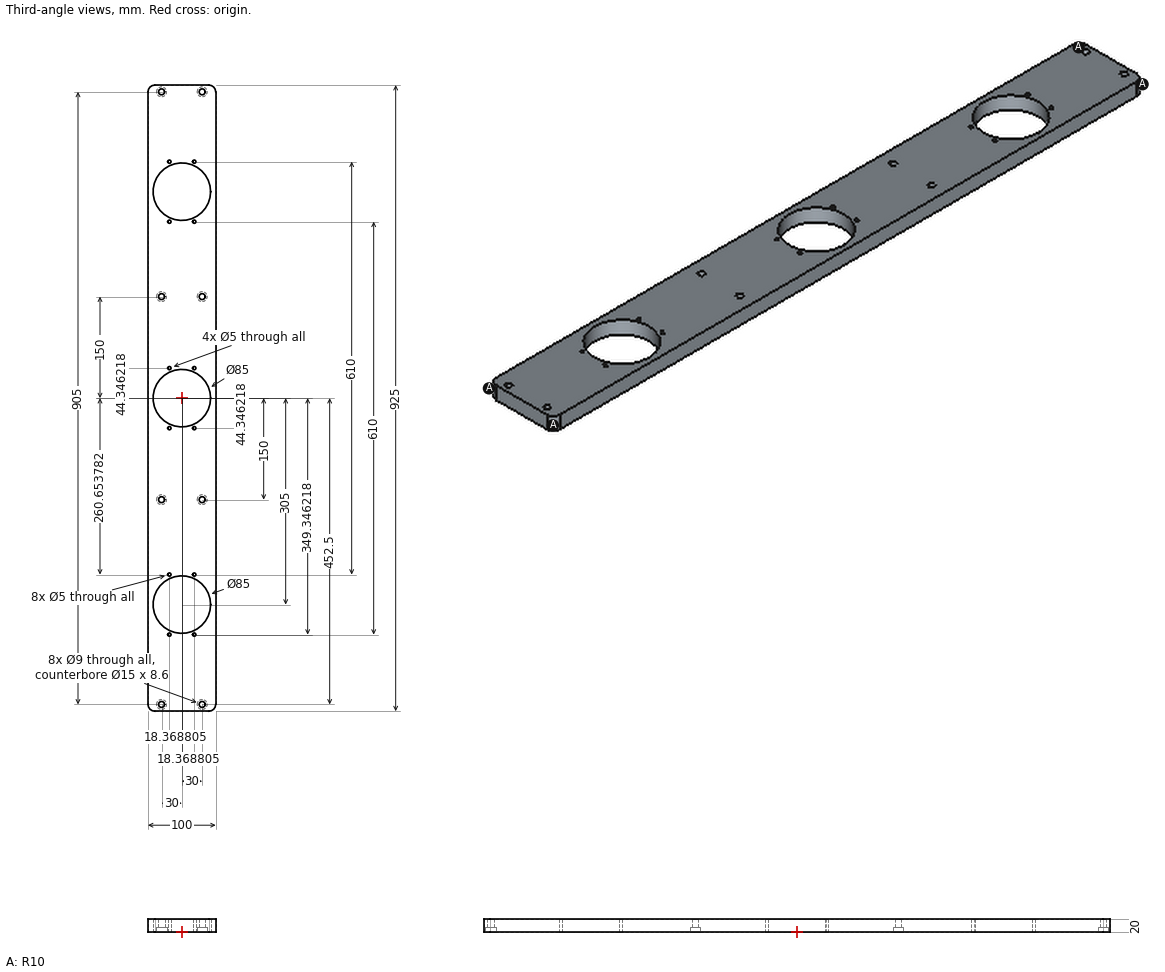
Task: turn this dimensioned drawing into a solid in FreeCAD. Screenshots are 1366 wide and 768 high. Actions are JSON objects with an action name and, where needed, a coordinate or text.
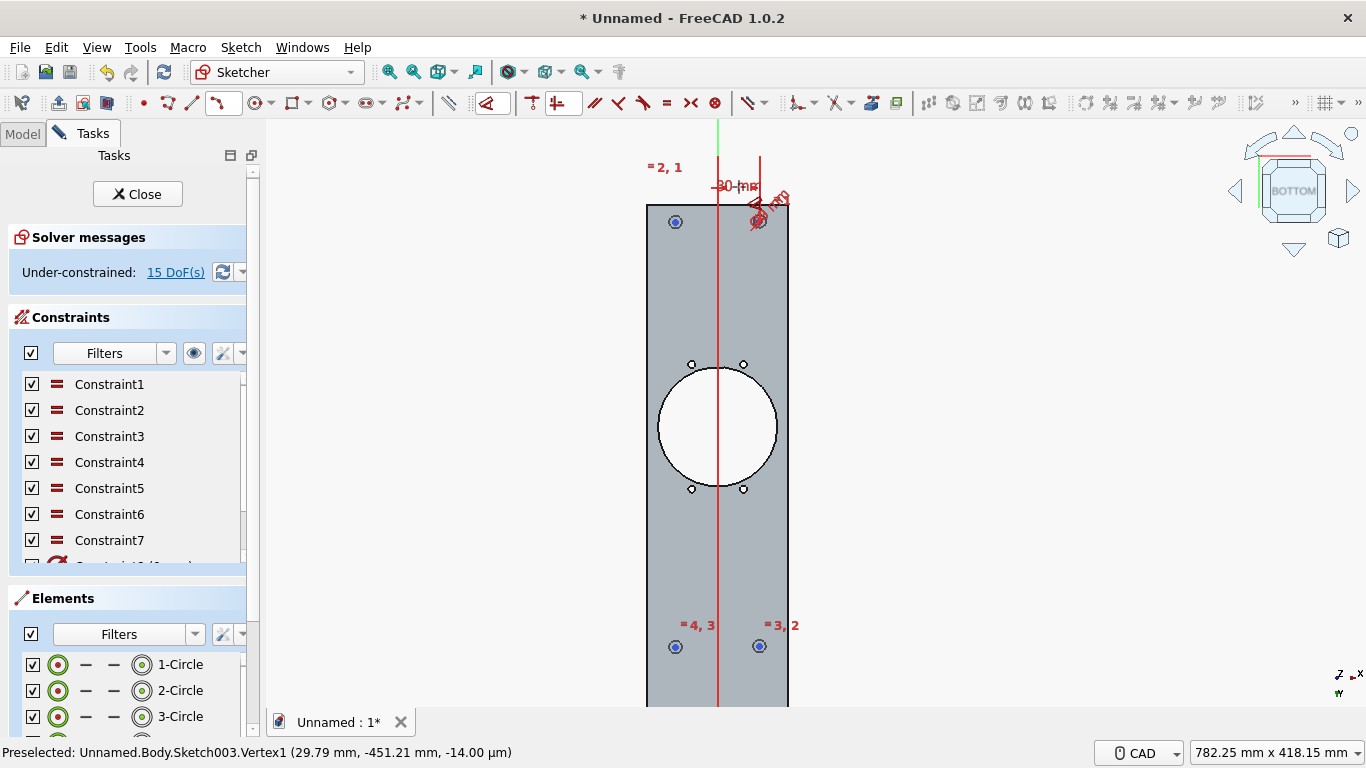
{"action": "left_click", "coordinate": [676, 222]}
{"action": "left_click", "coordinate": [697, 164]}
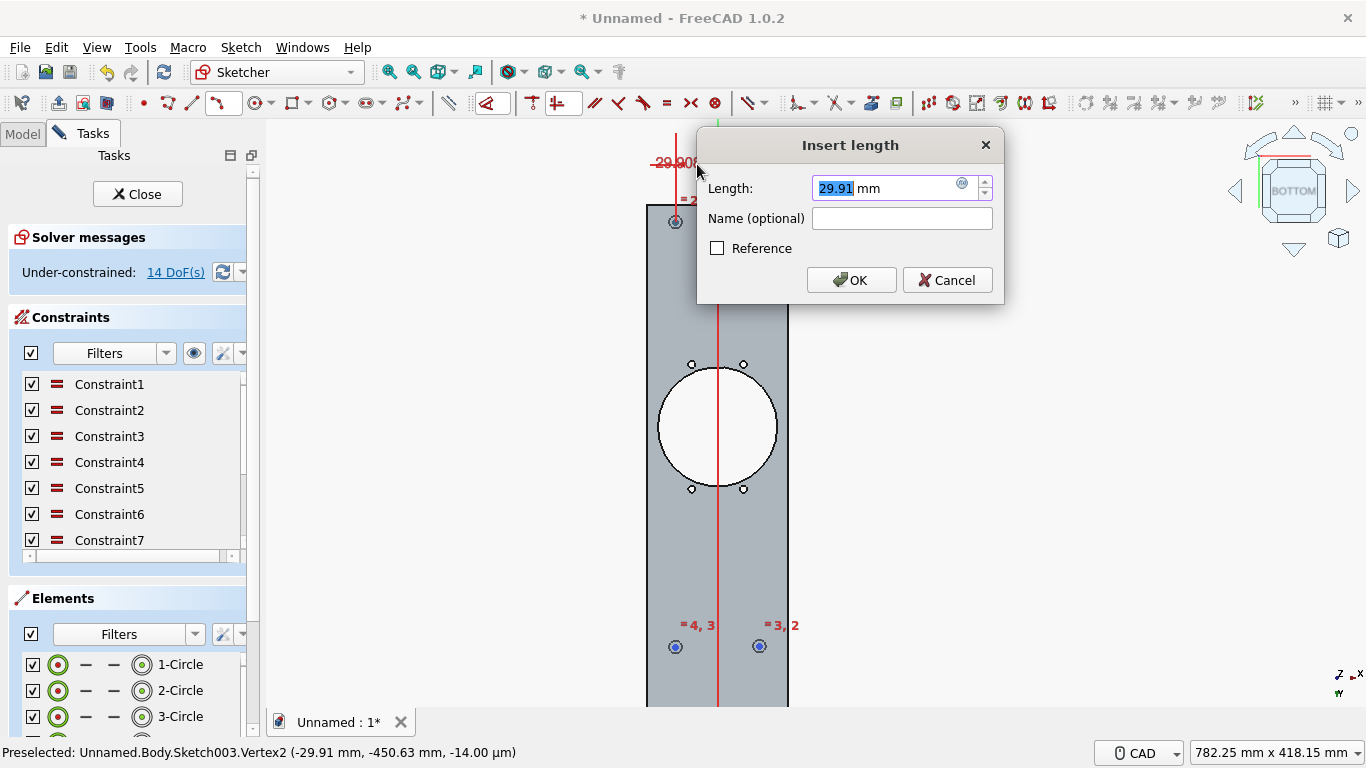
{"action": "type", "text": "30"}
{"action": "key", "text": "Return"}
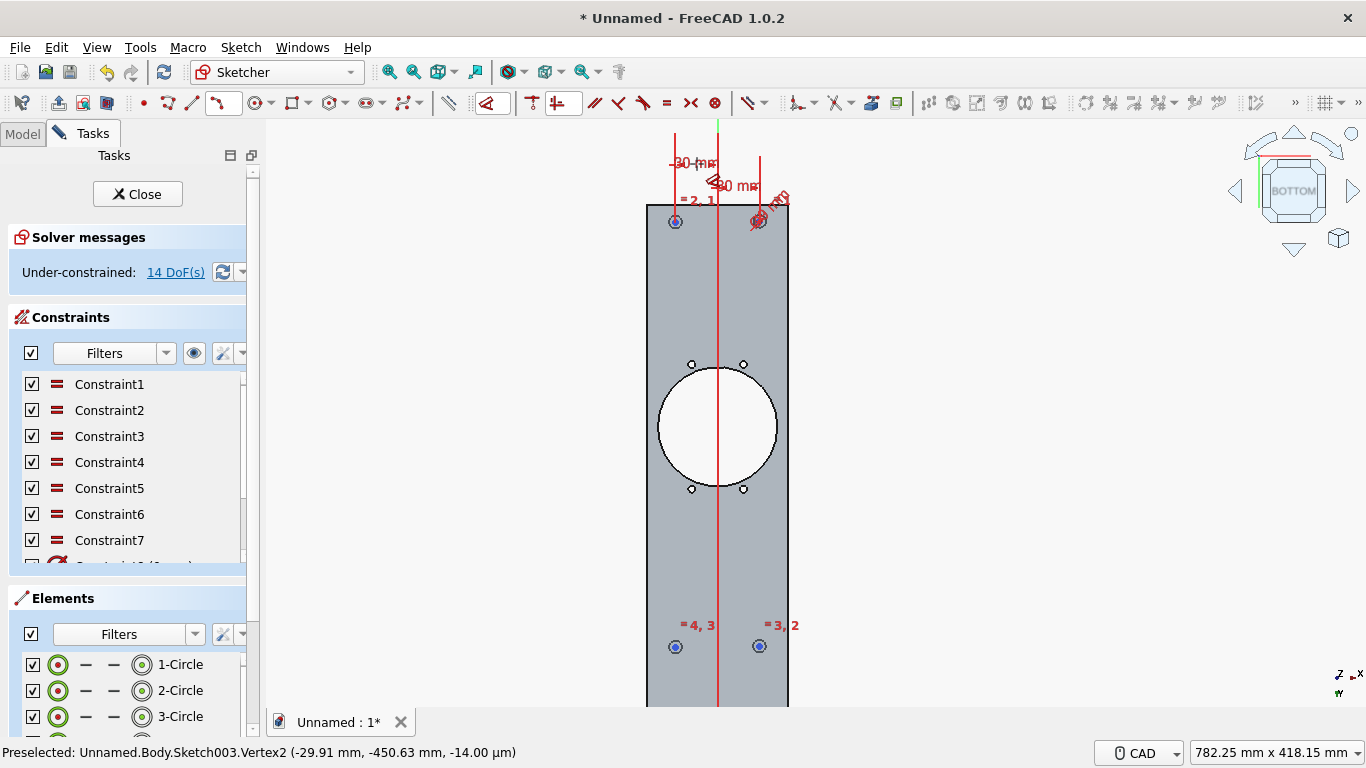
{"action": "left_click", "coordinate": [759, 646]}
{"action": "left_click", "coordinate": [739, 612]}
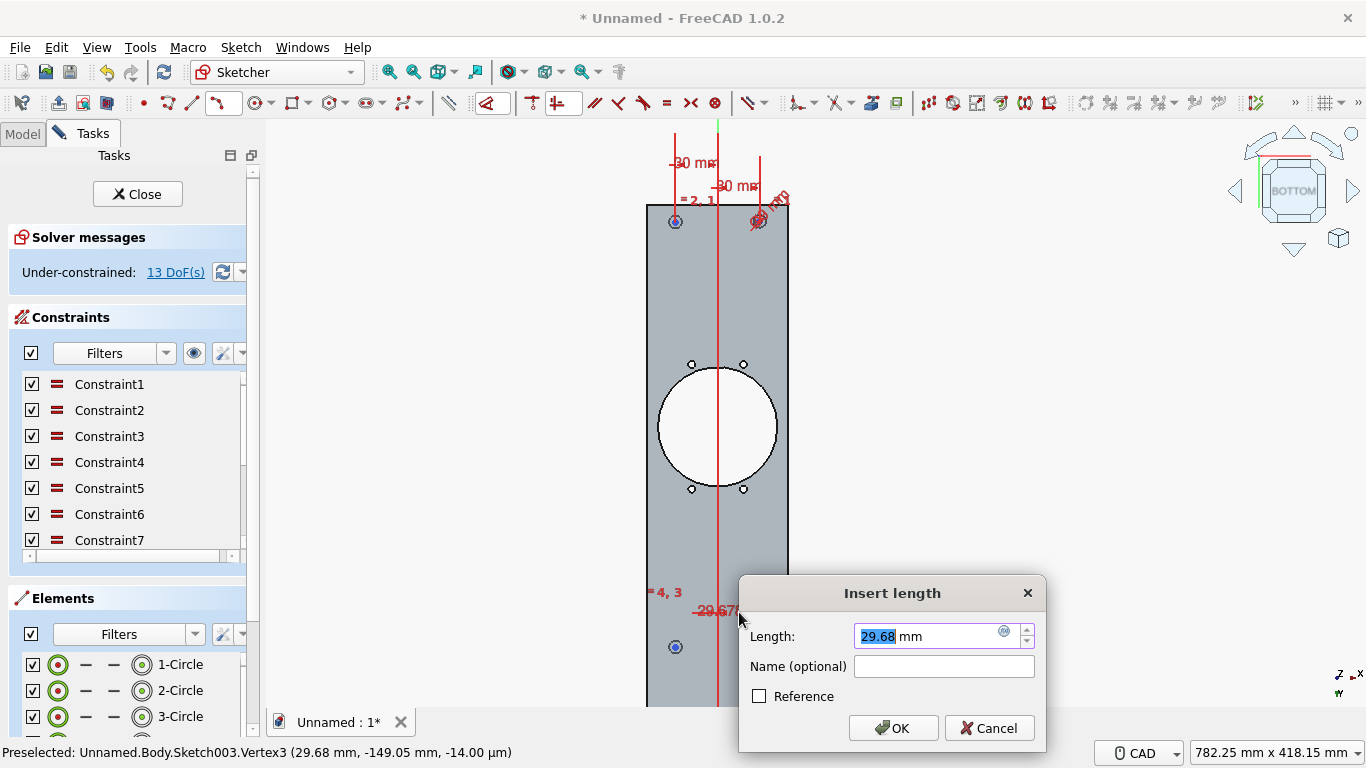
{"action": "type", "text": "30"}
{"action": "key", "text": "Return"}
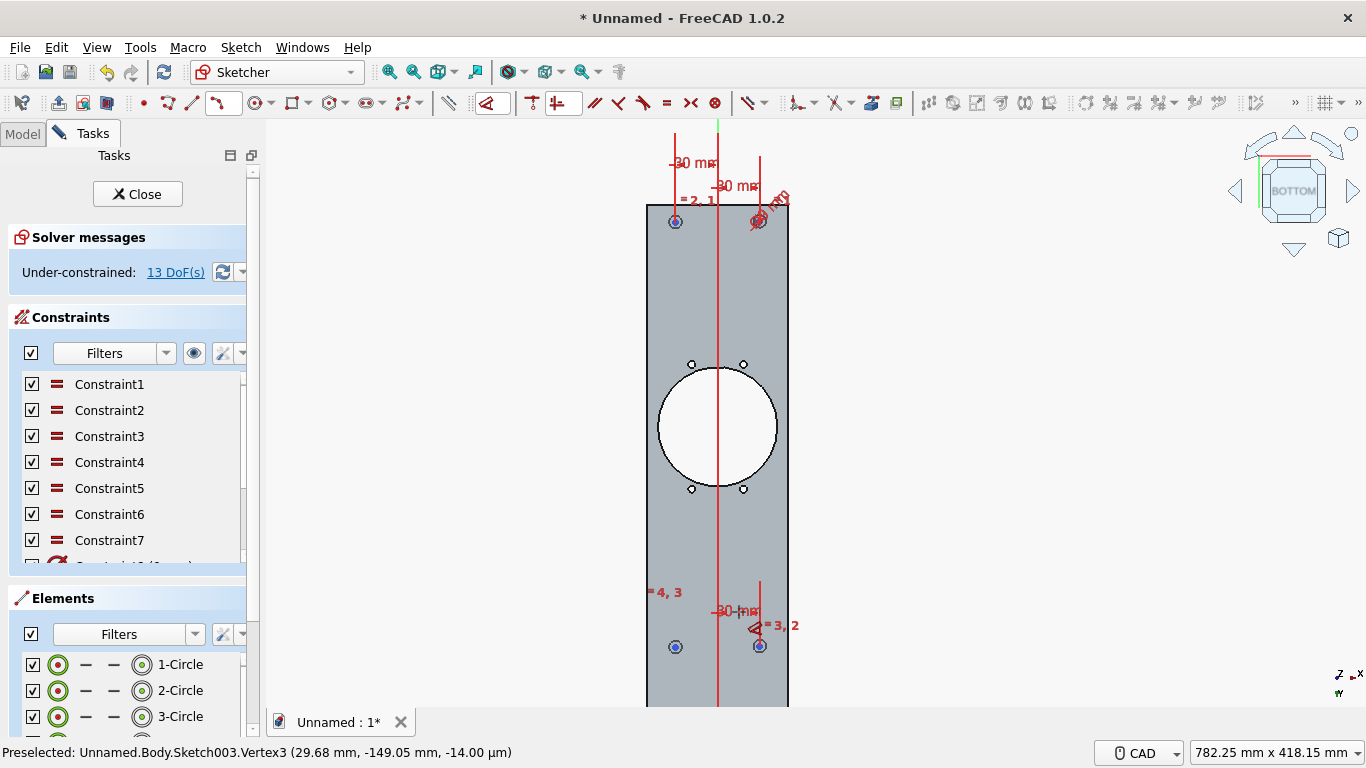
{"action": "left_click", "coordinate": [676, 647]}
{"action": "left_click", "coordinate": [697, 589]}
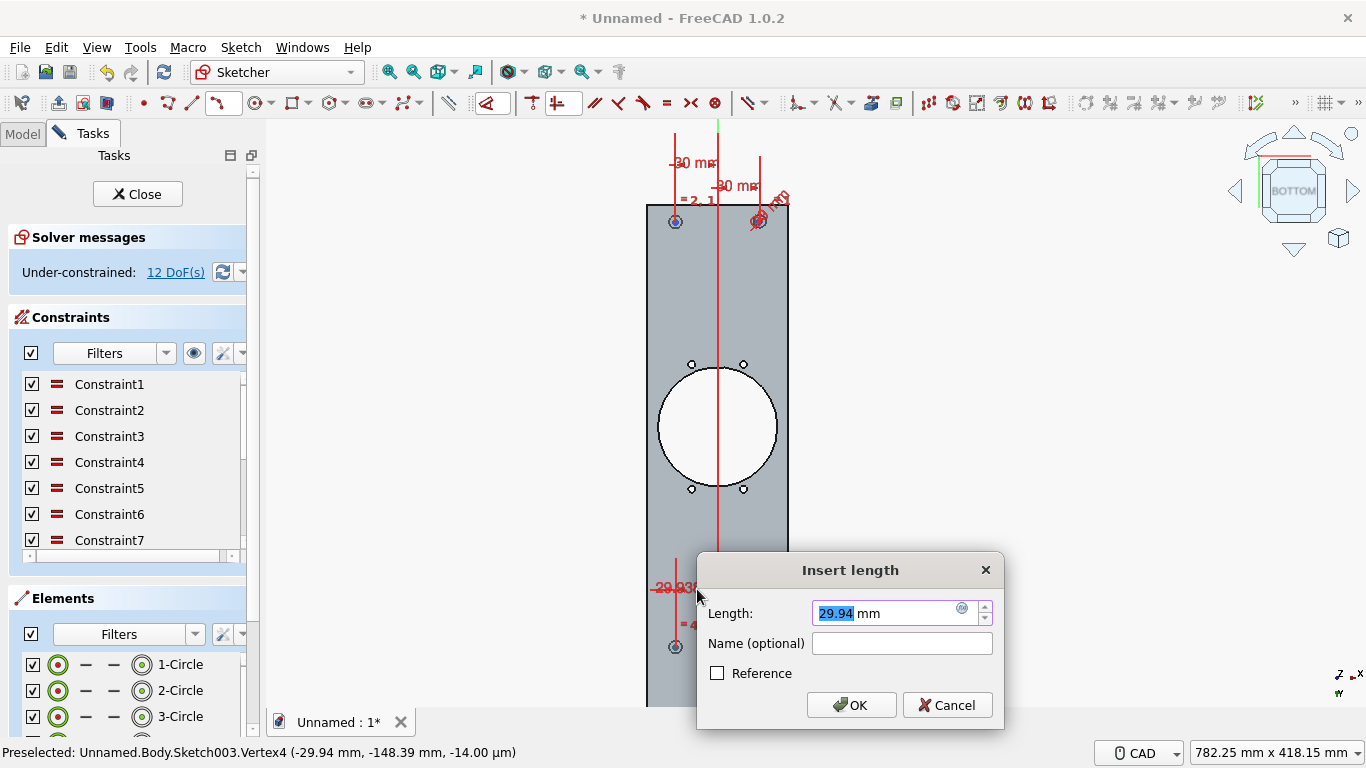
{"action": "type", "text": "30"}
{"action": "key", "text": "Return"}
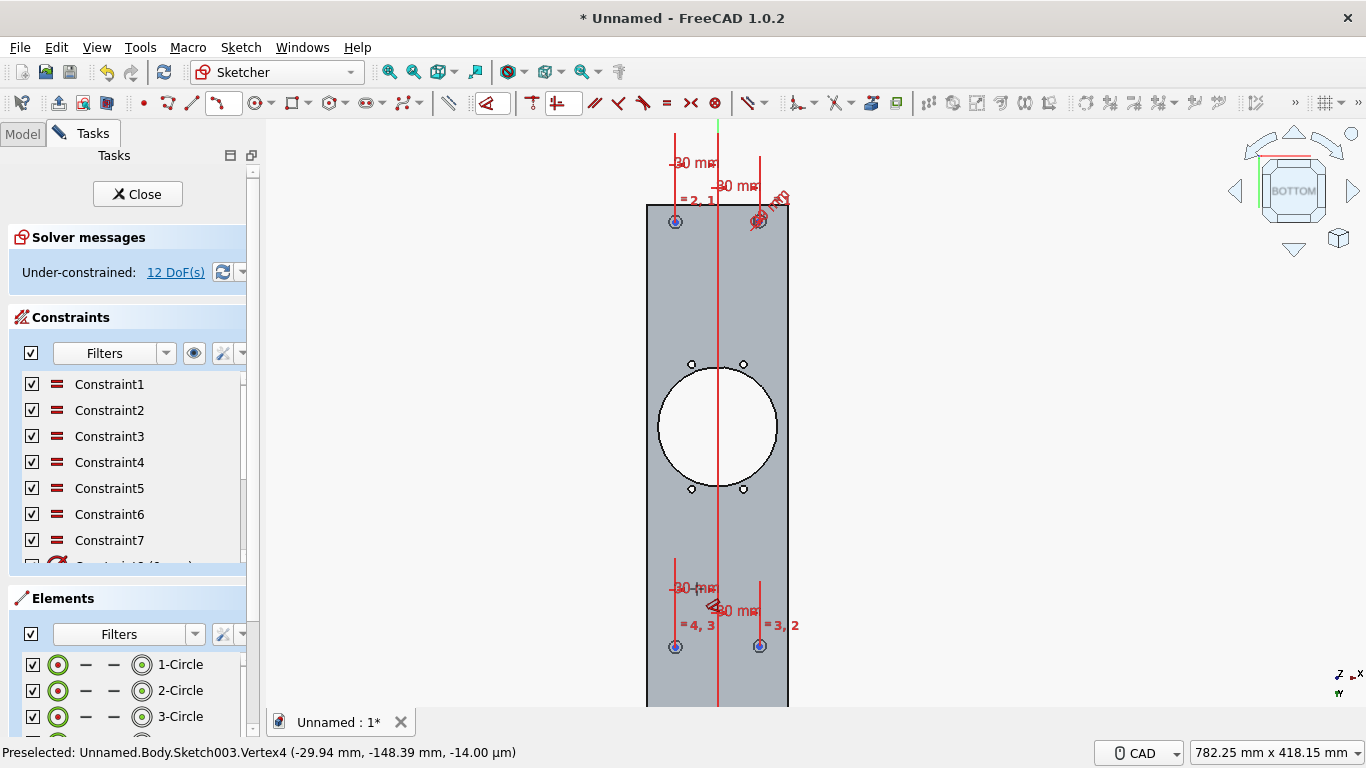
{"action": "scroll", "coordinate": [760, 222], "scroll_direction": "down", "scroll_amount": 6}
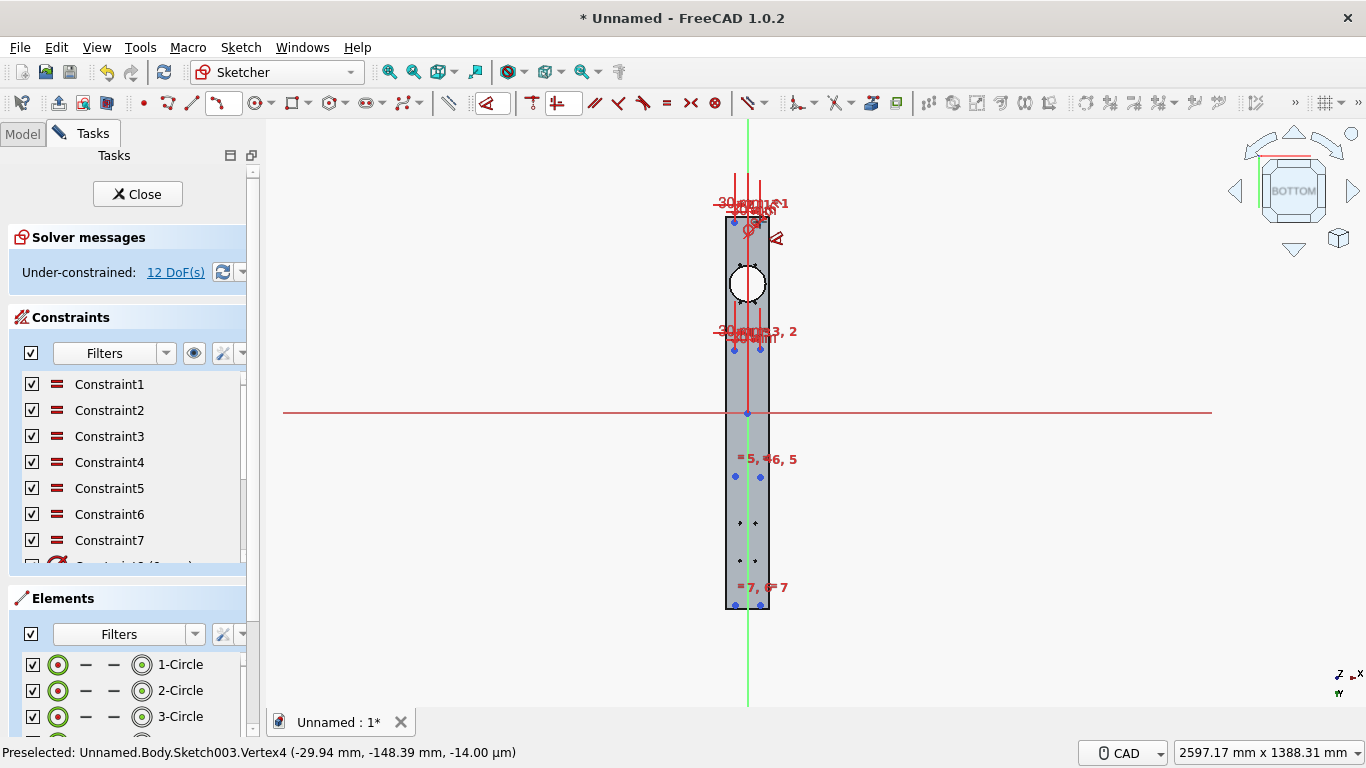
{"action": "scroll", "coordinate": [735, 477], "scroll_direction": "up", "scroll_amount": 6}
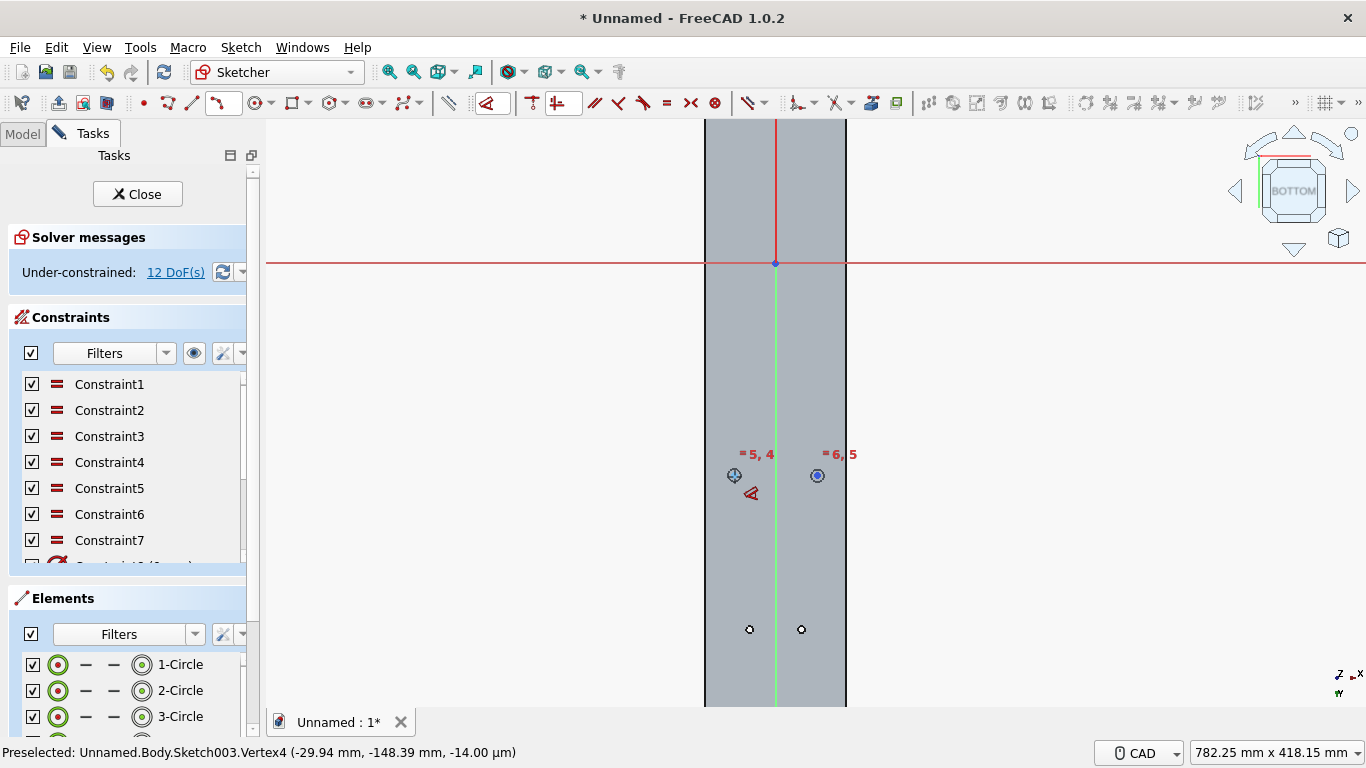
{"action": "left_click", "coordinate": [734, 475]}
{"action": "left_click", "coordinate": [755, 509]}